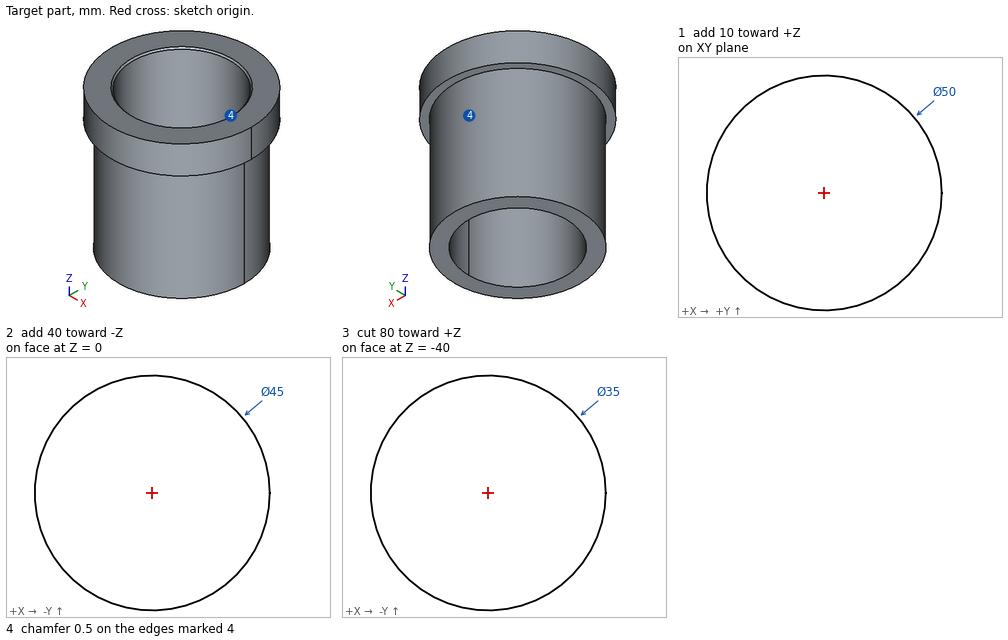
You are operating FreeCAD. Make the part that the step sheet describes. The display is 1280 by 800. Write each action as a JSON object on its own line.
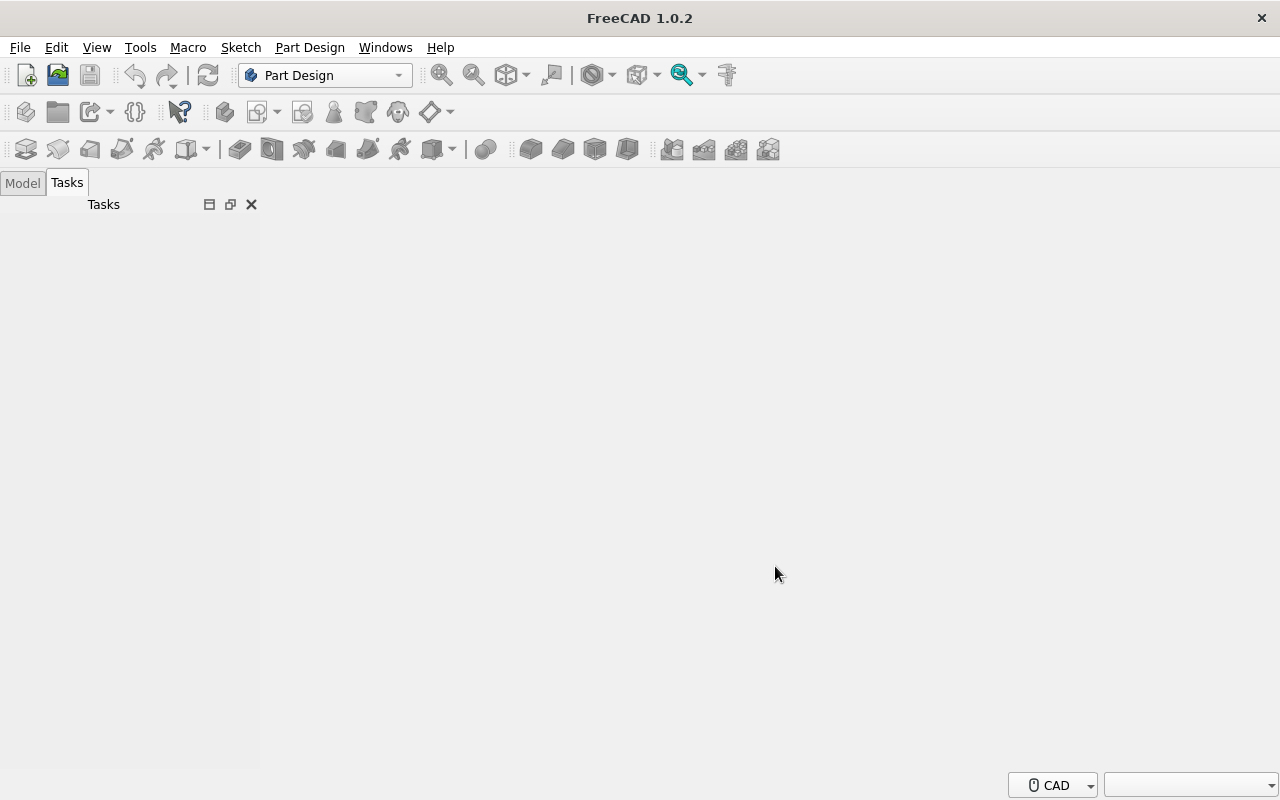
{"action": "key", "text": "ctrl+n"}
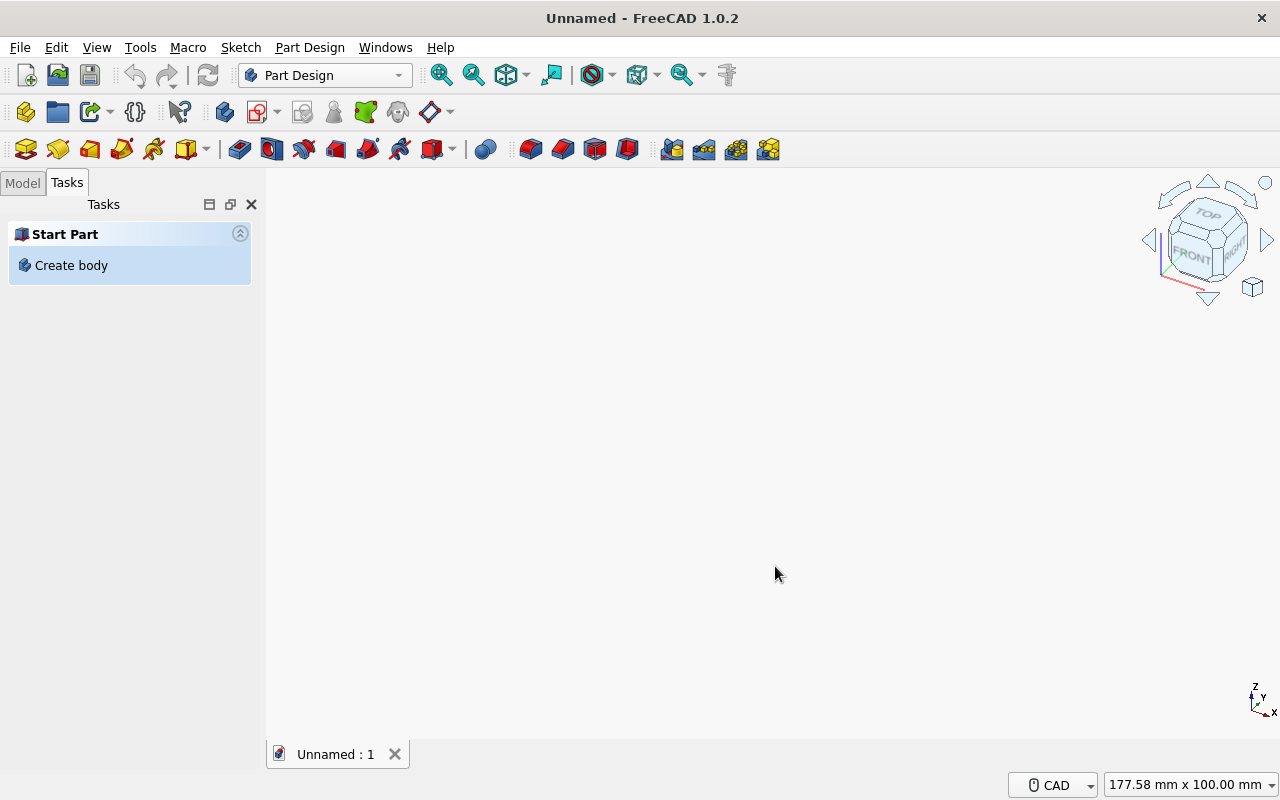
{"action": "left_click", "coordinate": [258, 112]}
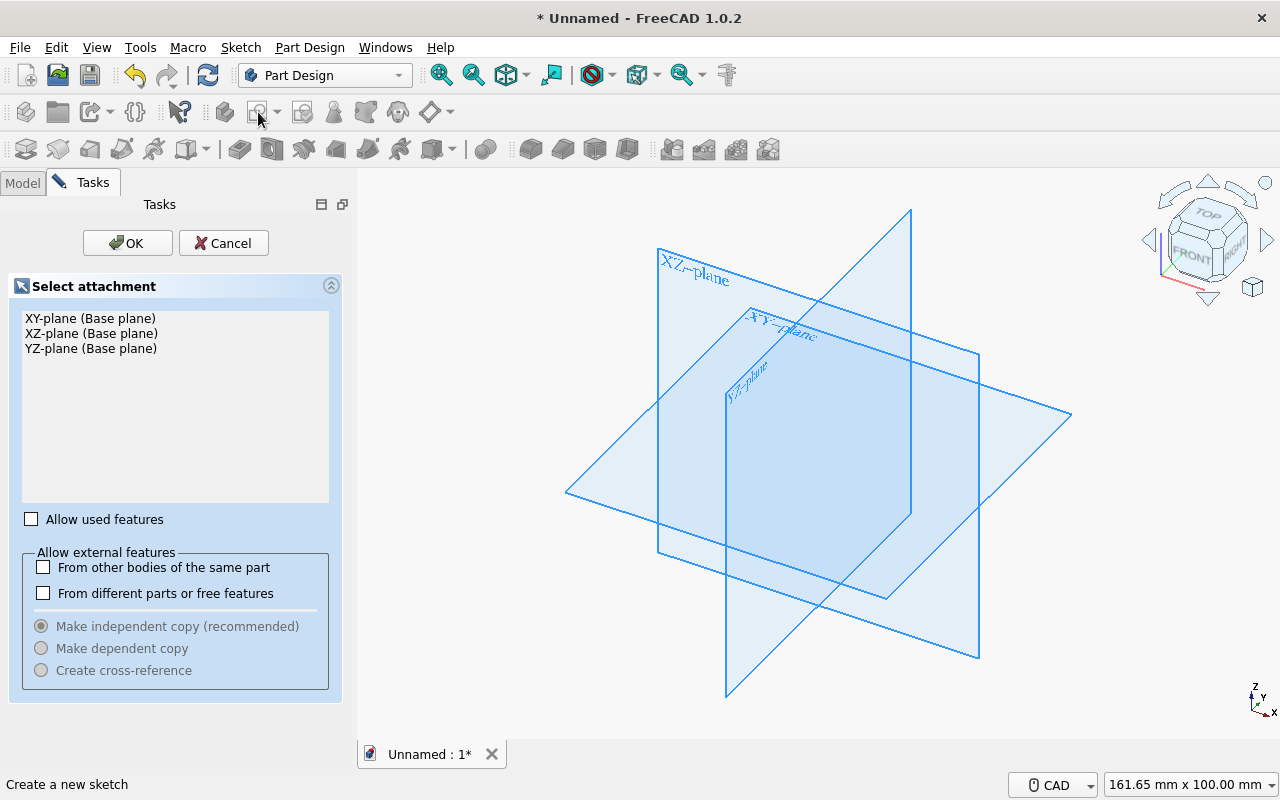
{"action": "left_click", "coordinate": [82, 318]}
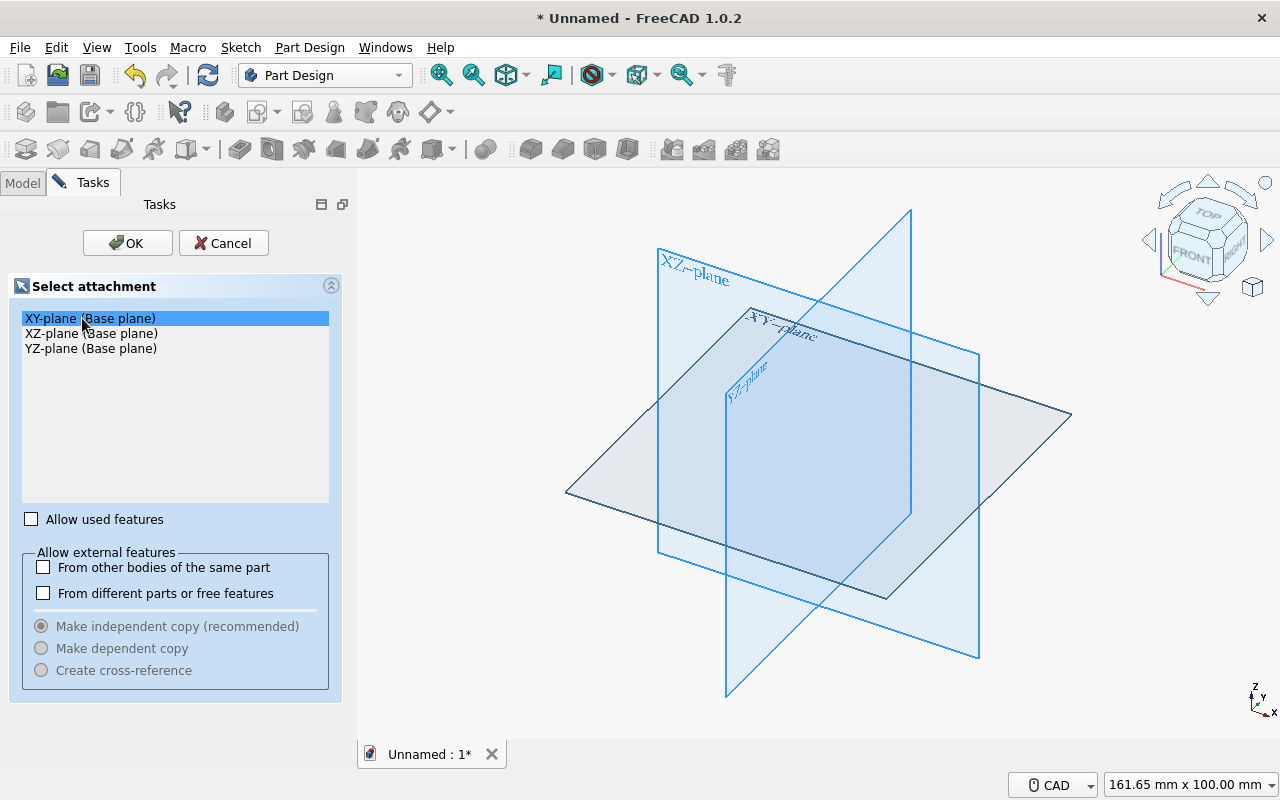
{"action": "left_click", "coordinate": [128, 243]}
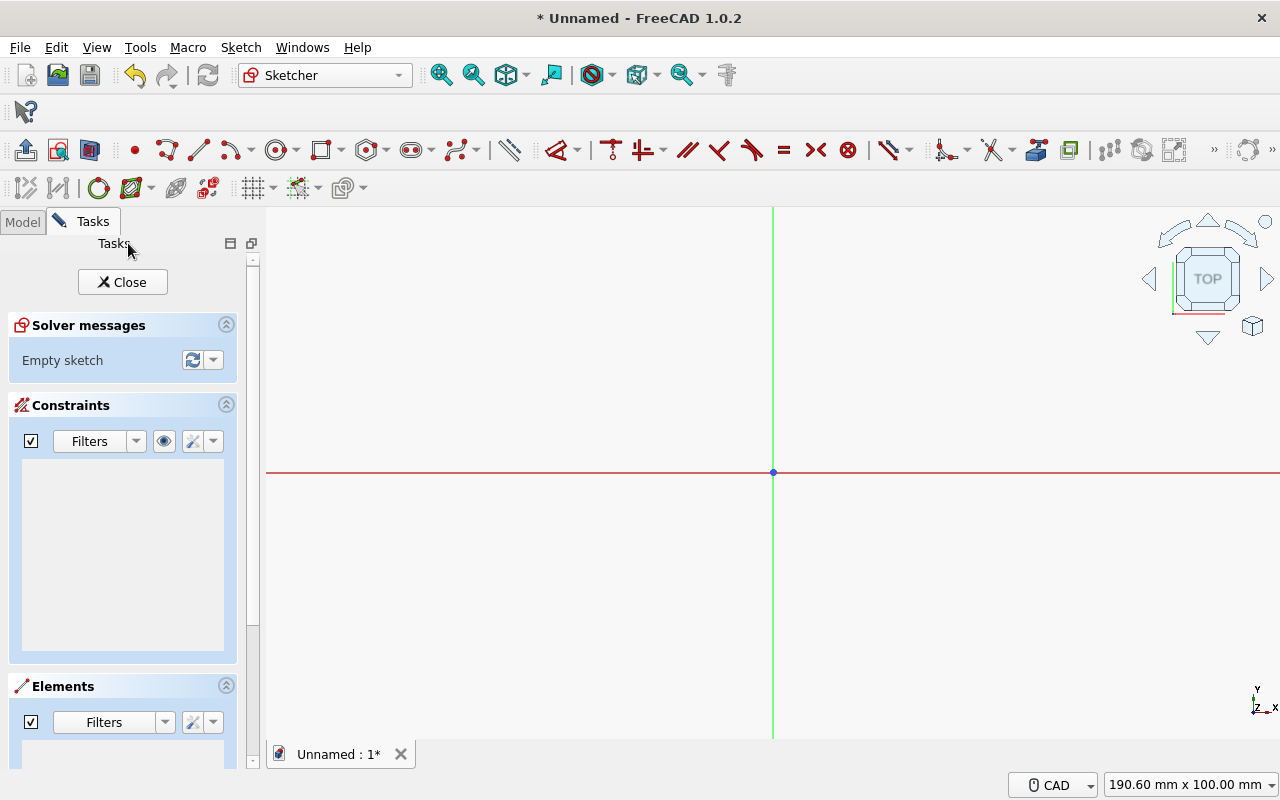
{"action": "key", "text": "g c"}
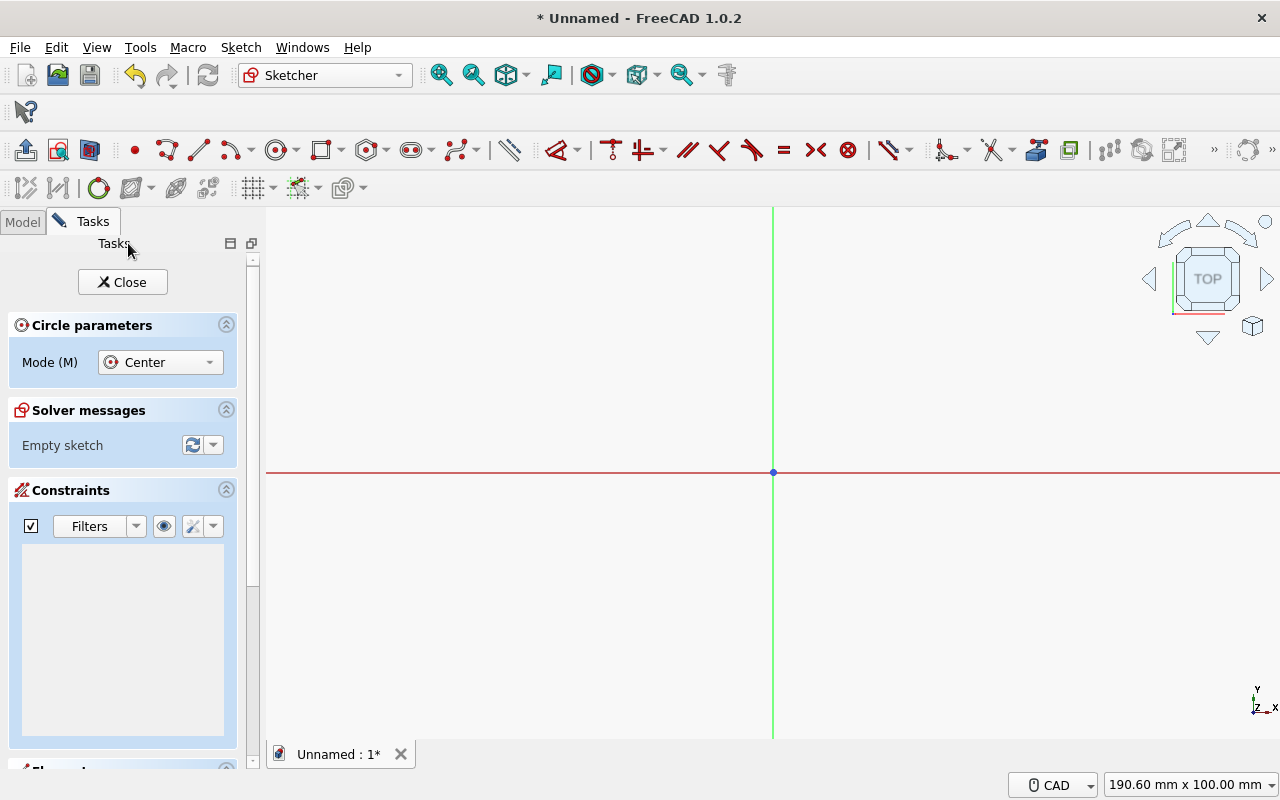
{"action": "left_click", "coordinate": [773, 473]}
{"action": "left_click", "coordinate": [867, 379]}
{"action": "key", "text": "Escape"}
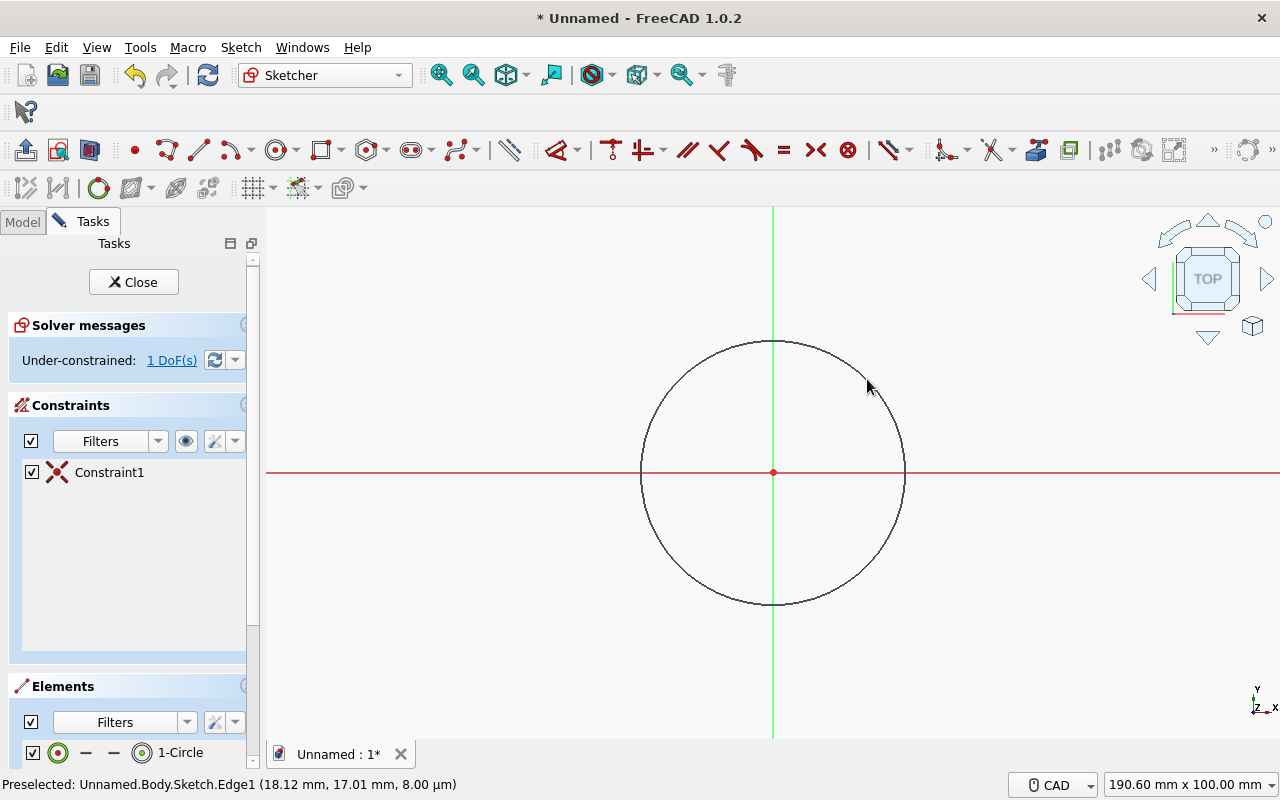
{"action": "key", "text": "d"}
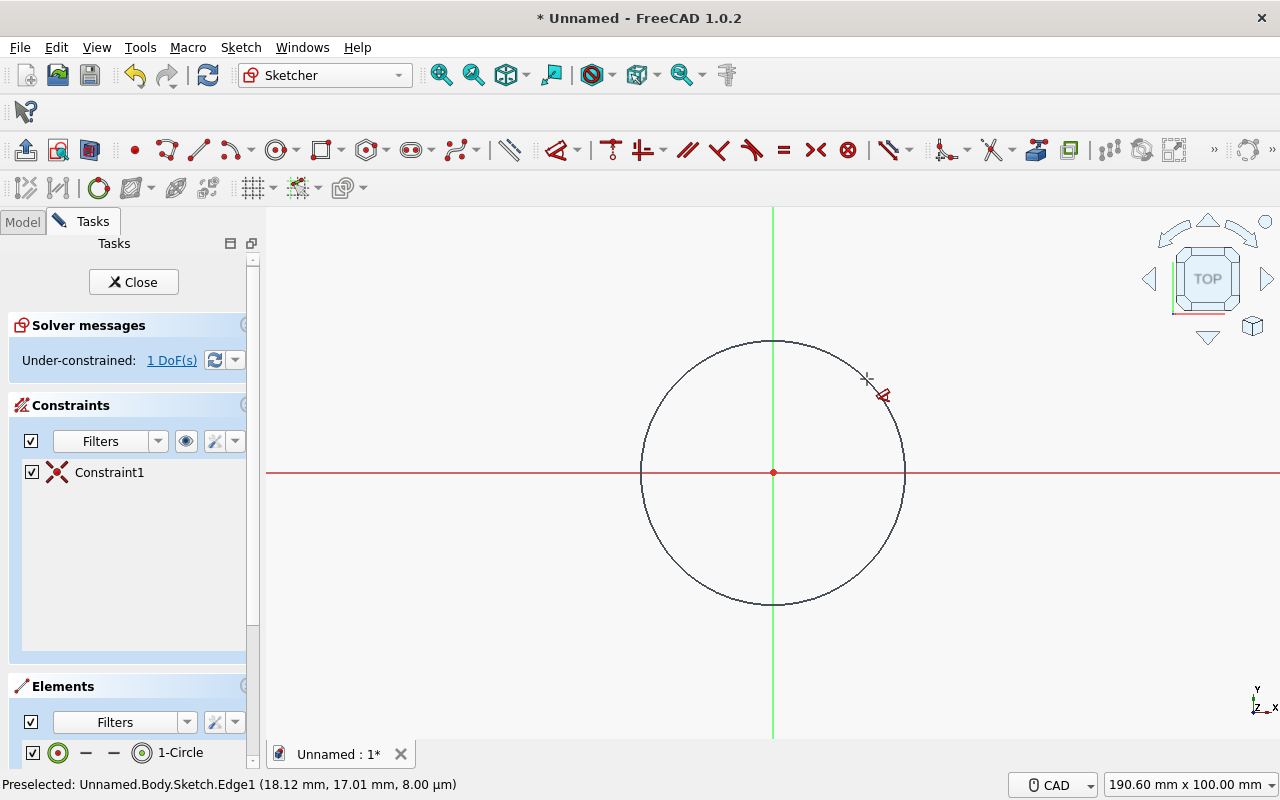
{"action": "left_click", "coordinate": [866, 379]}
{"action": "left_click", "coordinate": [889, 356]}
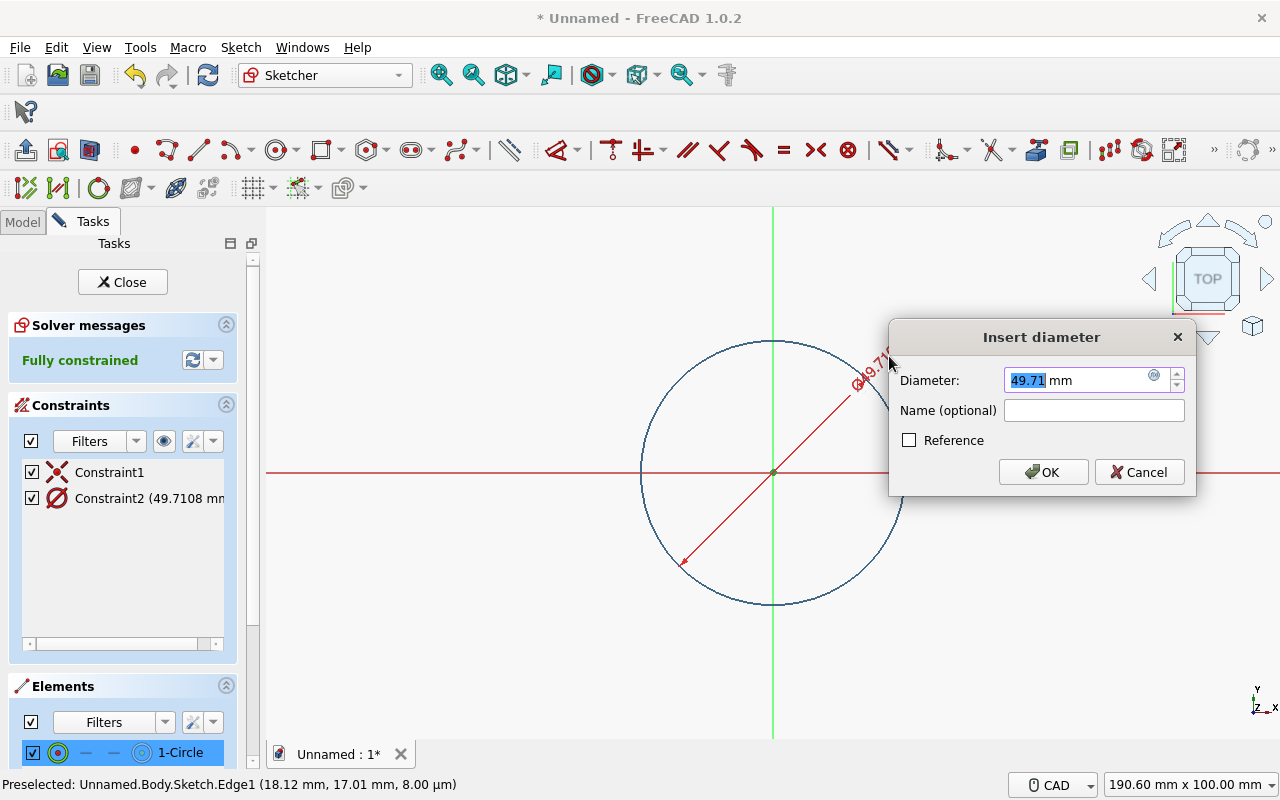
{"action": "type", "text": "50"}
{"action": "key", "text": "Return"}
{"action": "key", "text": "Escape"}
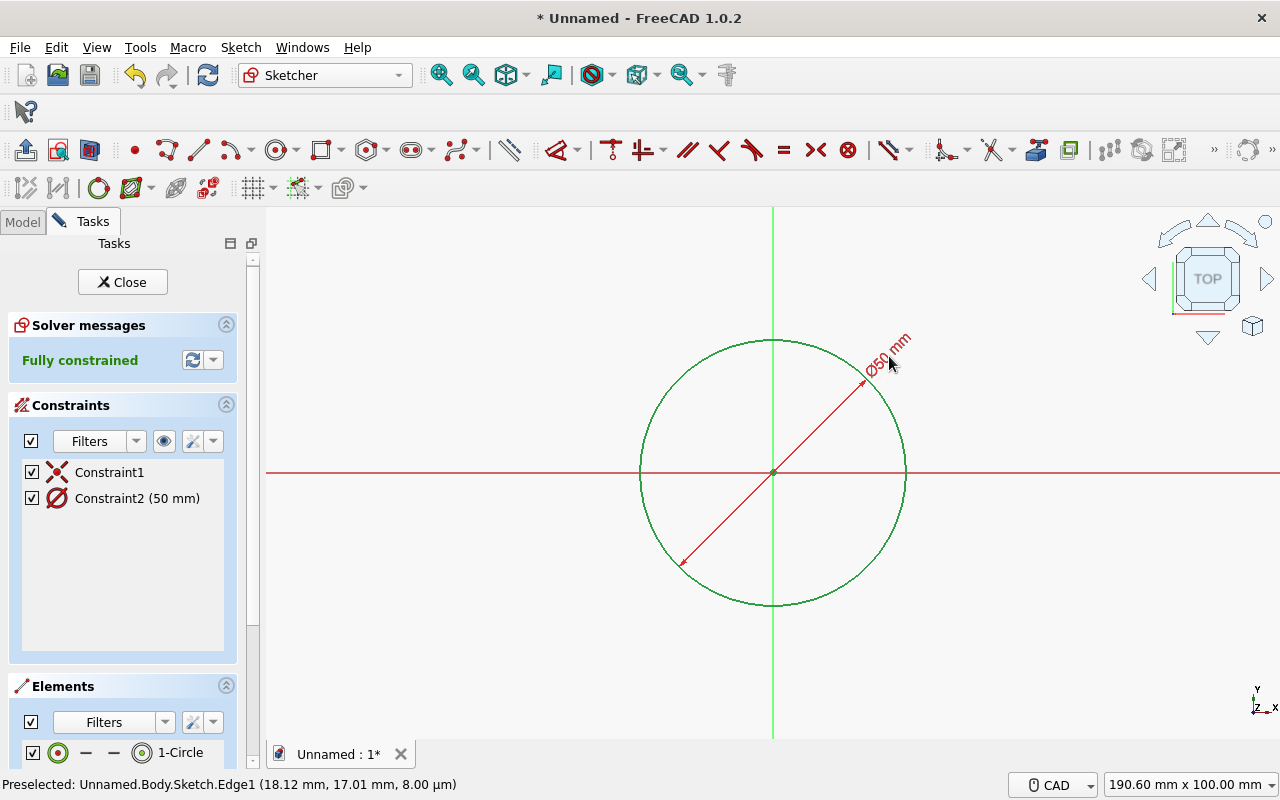
{"action": "left_click", "coordinate": [123, 282]}